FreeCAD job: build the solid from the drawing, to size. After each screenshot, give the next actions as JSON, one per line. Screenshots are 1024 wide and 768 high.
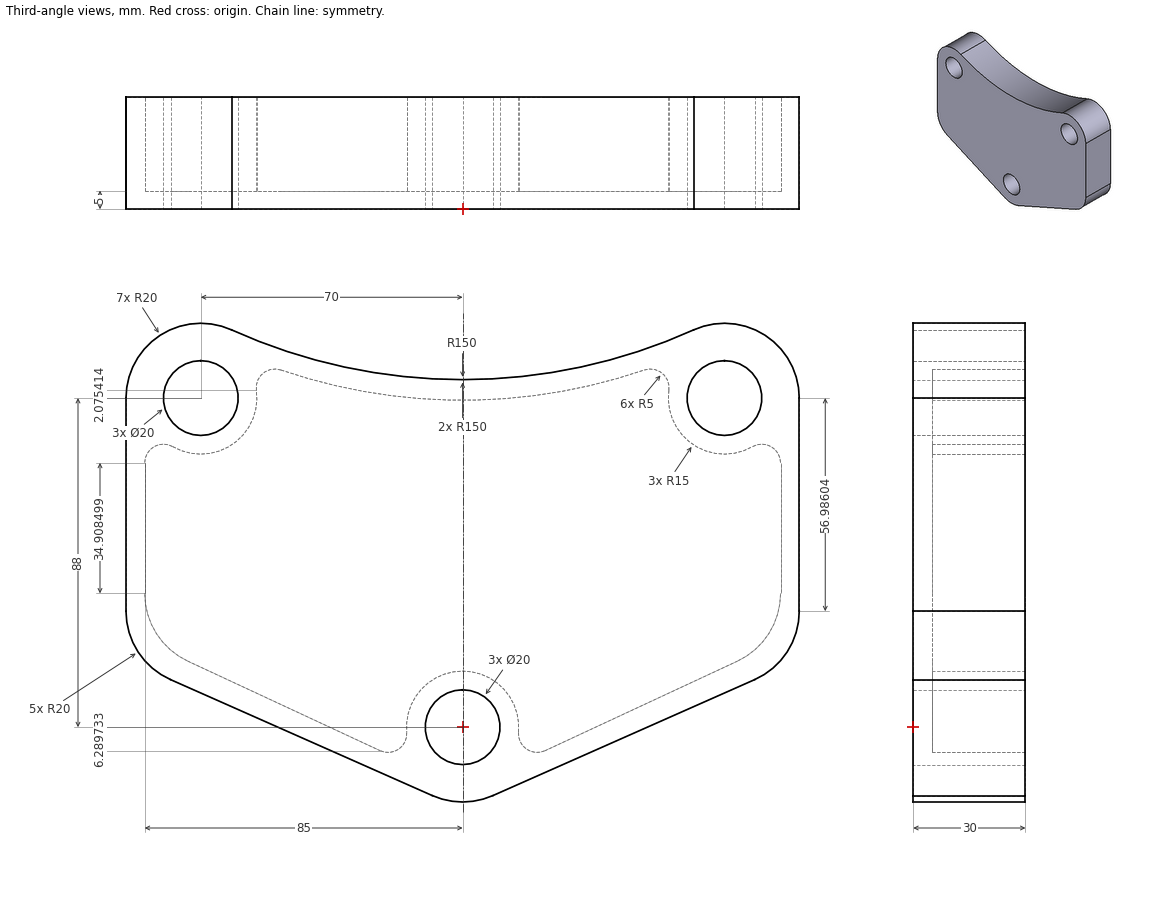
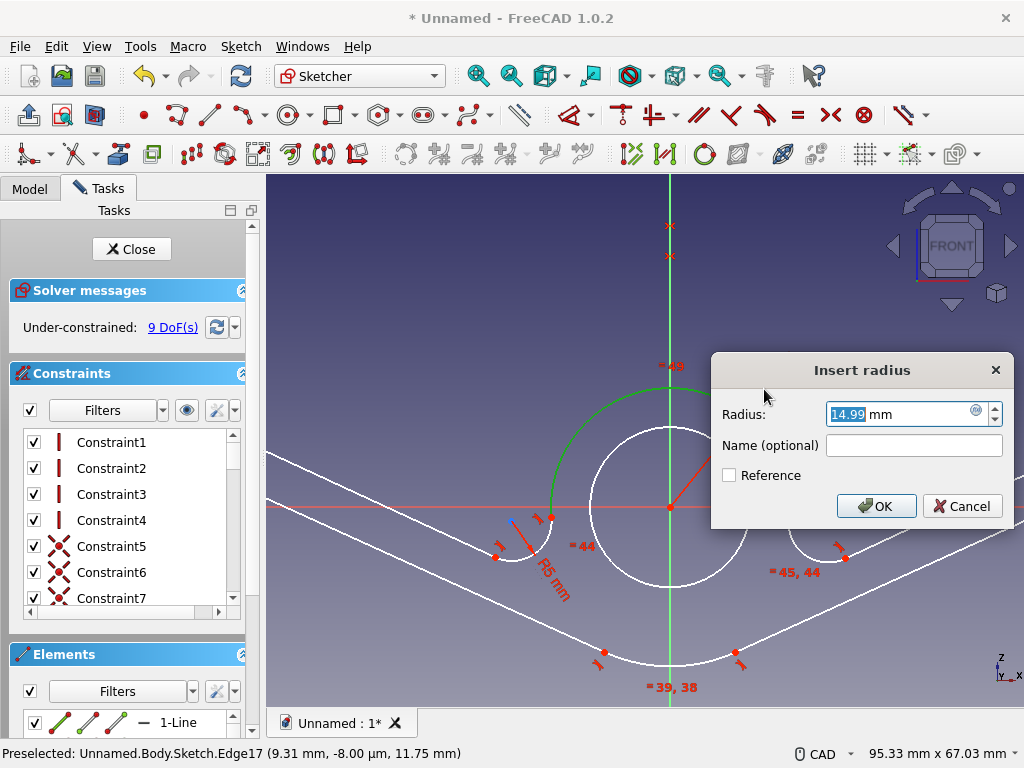
{"action": "type", "text": "15"}
{"action": "key", "text": "Return"}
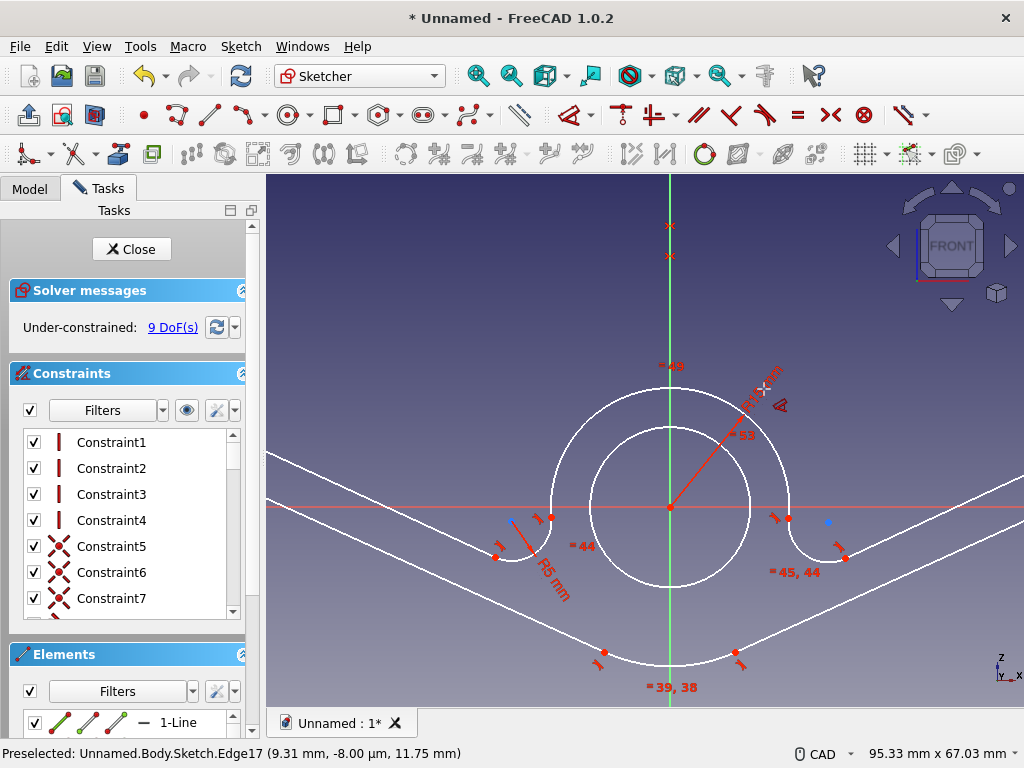
{"action": "scroll", "coordinate": [536, 559], "scroll_direction": "down", "scroll_amount": 6}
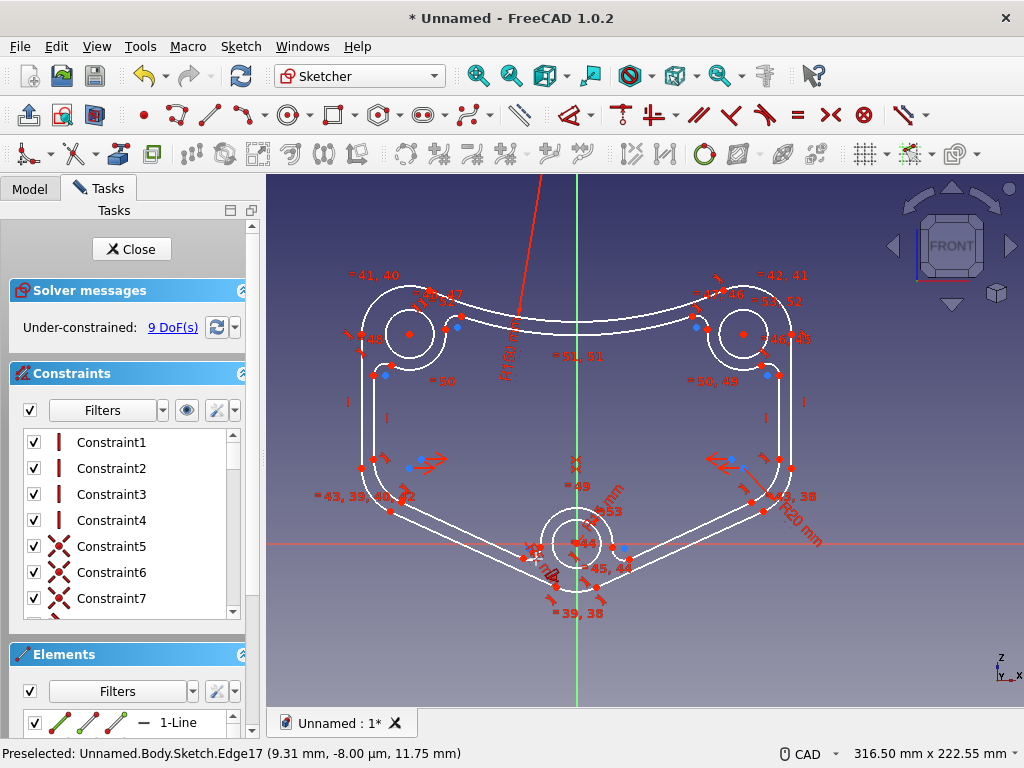
{"action": "left_click", "coordinate": [427, 317]}
{"action": "left_click", "coordinate": [449, 374]}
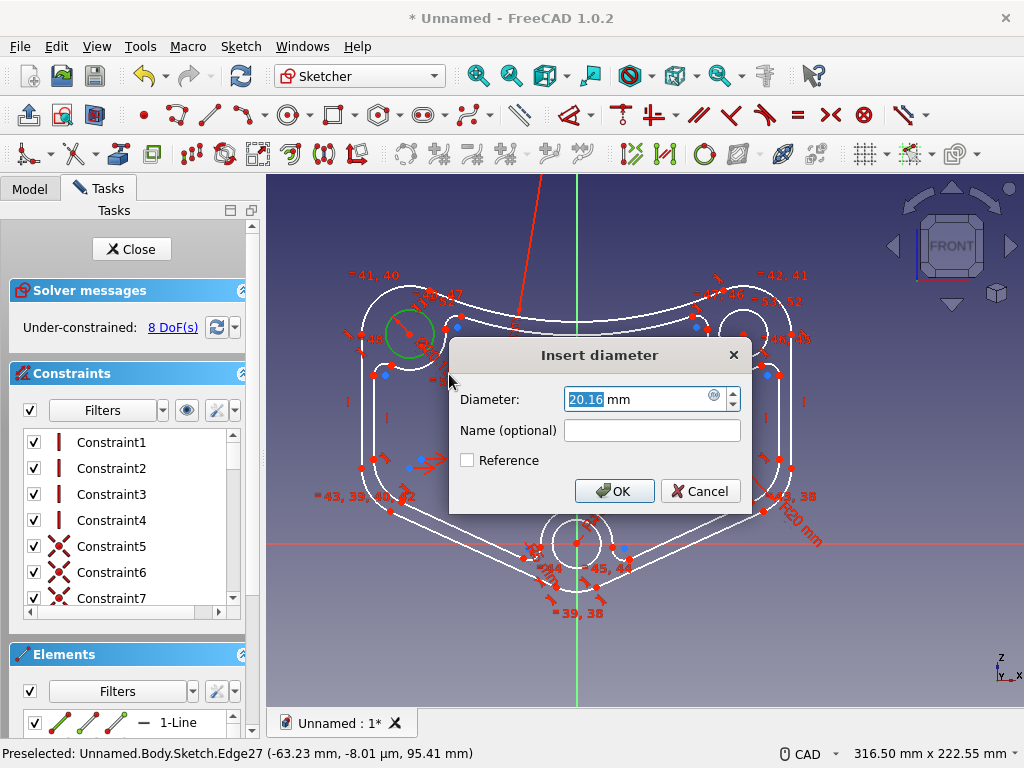
{"action": "type", "text": "20"}
{"action": "key", "text": "Return"}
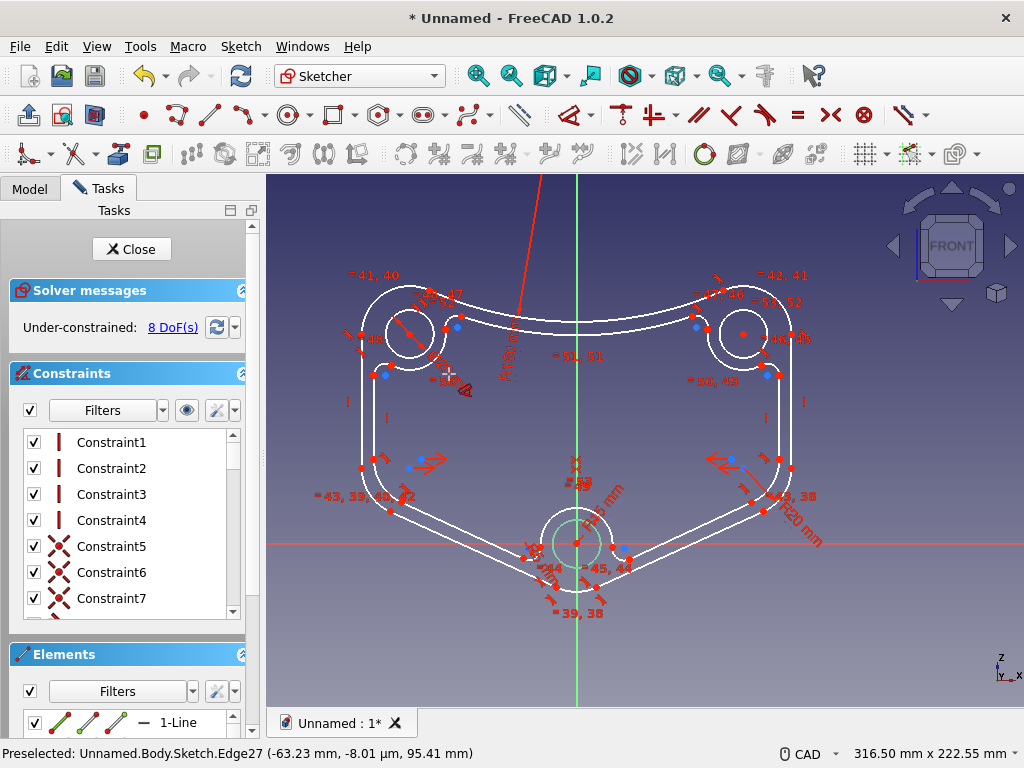
{"action": "left_click", "coordinate": [410, 334]}
{"action": "left_click", "coordinate": [532, 300]}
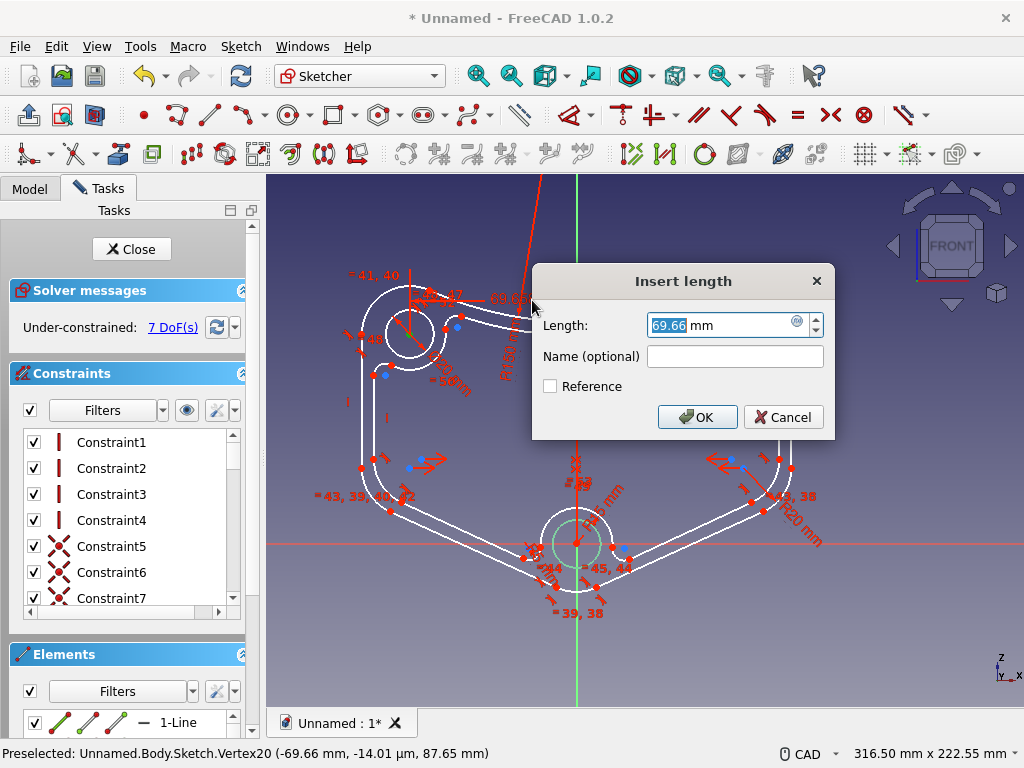
{"action": "type", "text": "70"}
{"action": "key", "text": "Return"}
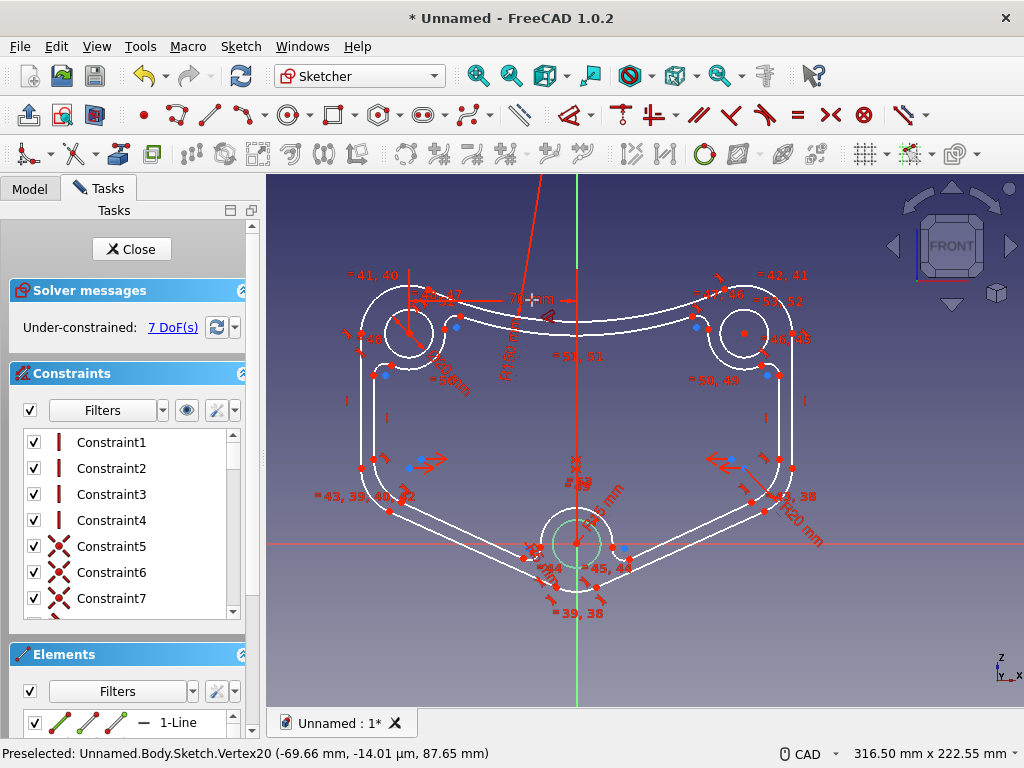
{"action": "left_click", "coordinate": [409, 334]}
{"action": "left_click", "coordinate": [611, 439]}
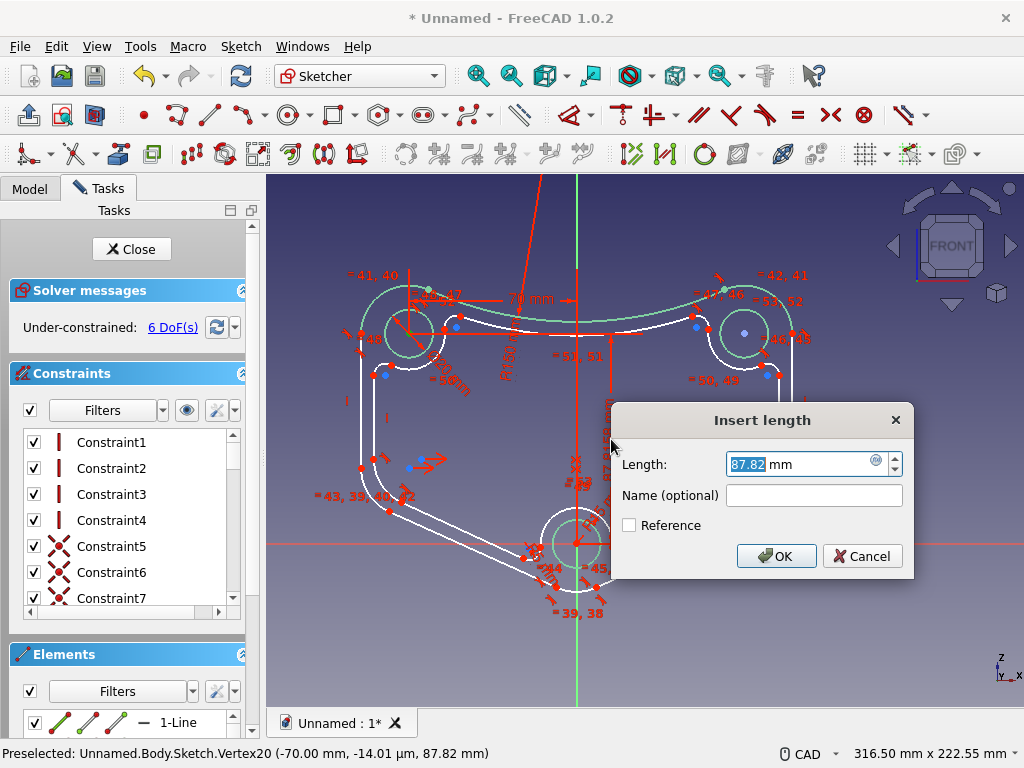
{"action": "type", "text": "88"}
{"action": "key", "text": "Return"}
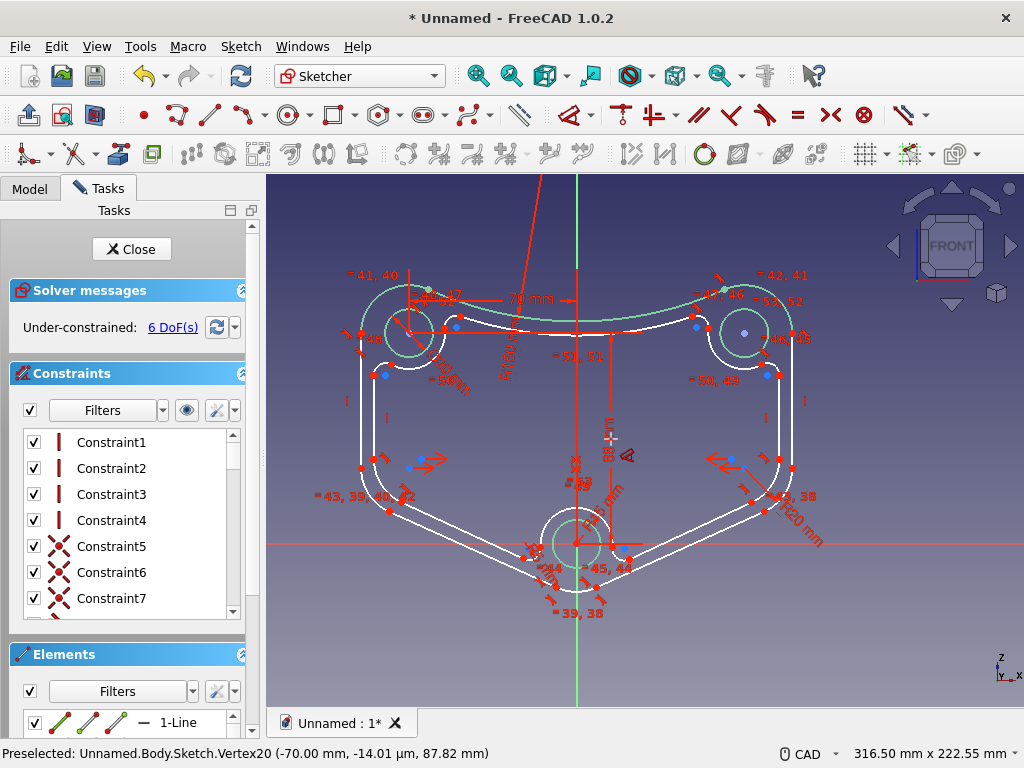
{"action": "left_click", "coordinate": [374, 375]}
{"action": "left_click", "coordinate": [429, 578]}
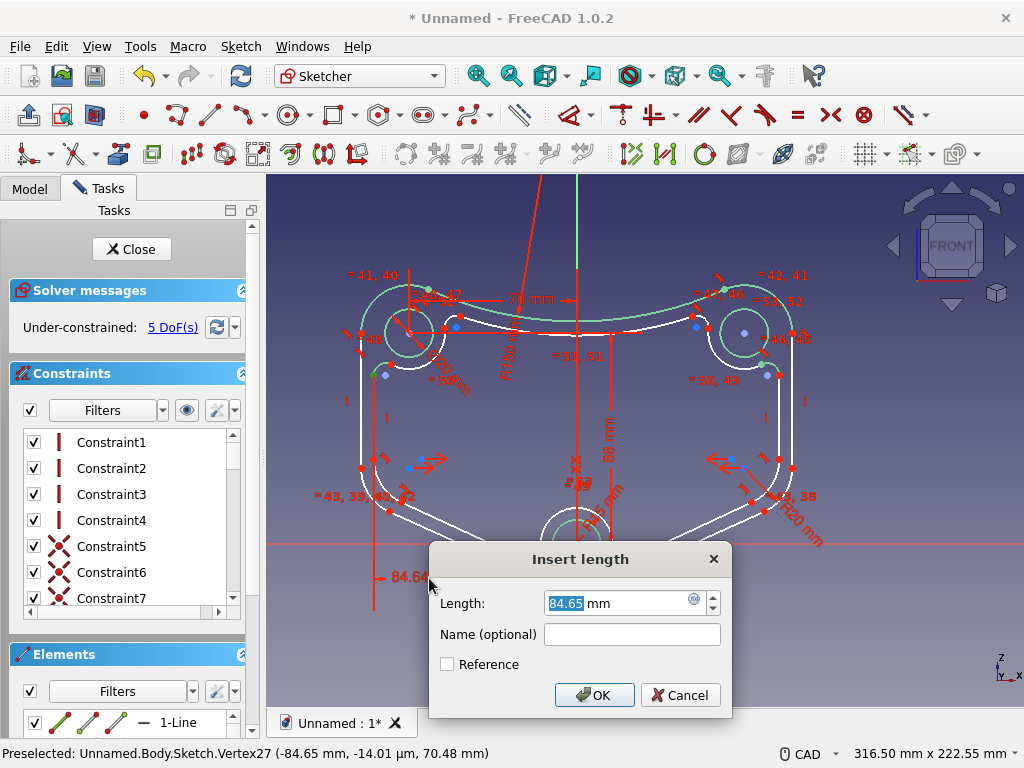
{"action": "type", "text": "85"}
{"action": "key", "text": "Return"}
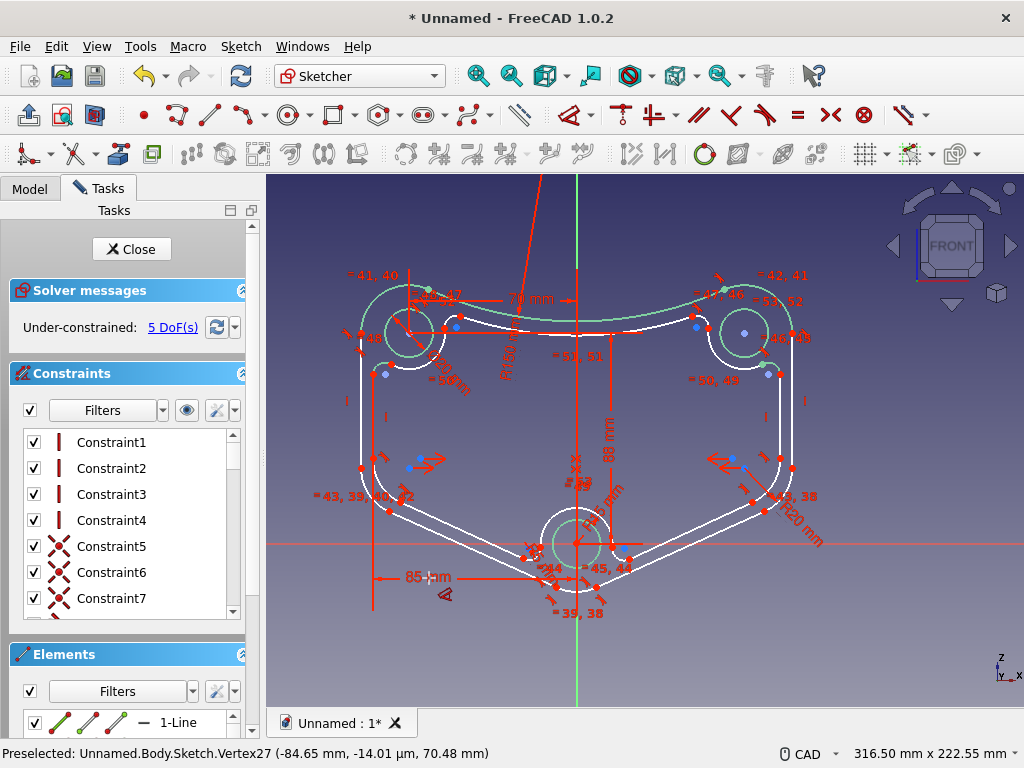
{"action": "left_click", "coordinate": [792, 374]}
{"action": "left_click", "coordinate": [826, 401]}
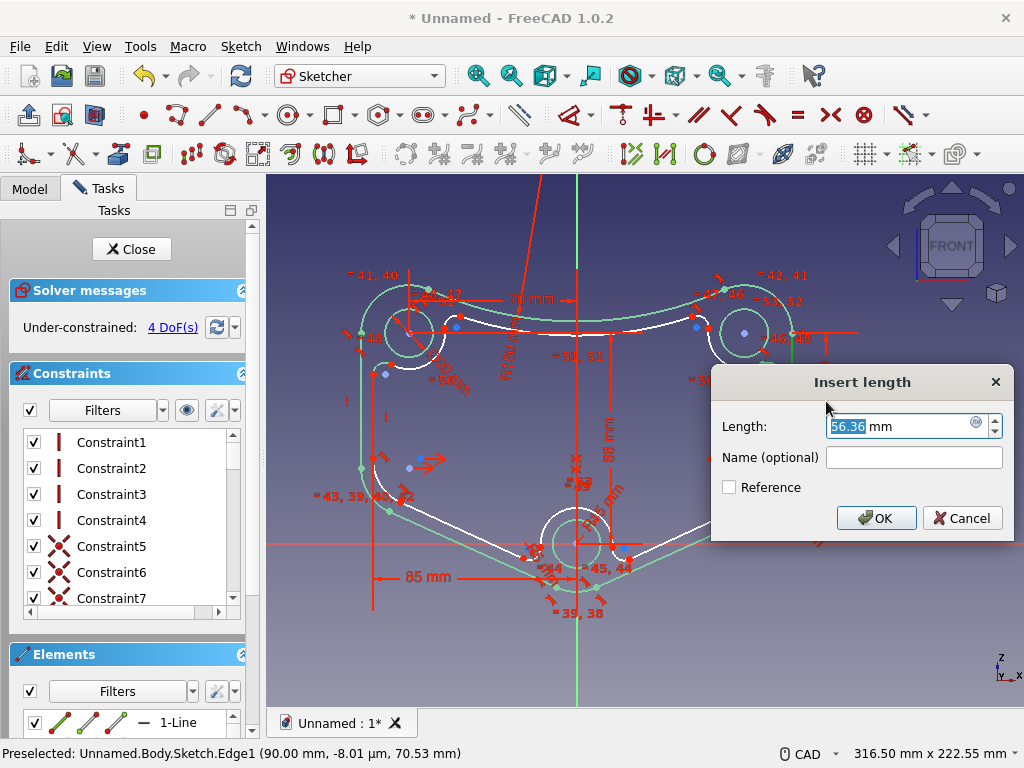
{"action": "type", "text": "56.98604"}
{"action": "key", "text": "Return"}